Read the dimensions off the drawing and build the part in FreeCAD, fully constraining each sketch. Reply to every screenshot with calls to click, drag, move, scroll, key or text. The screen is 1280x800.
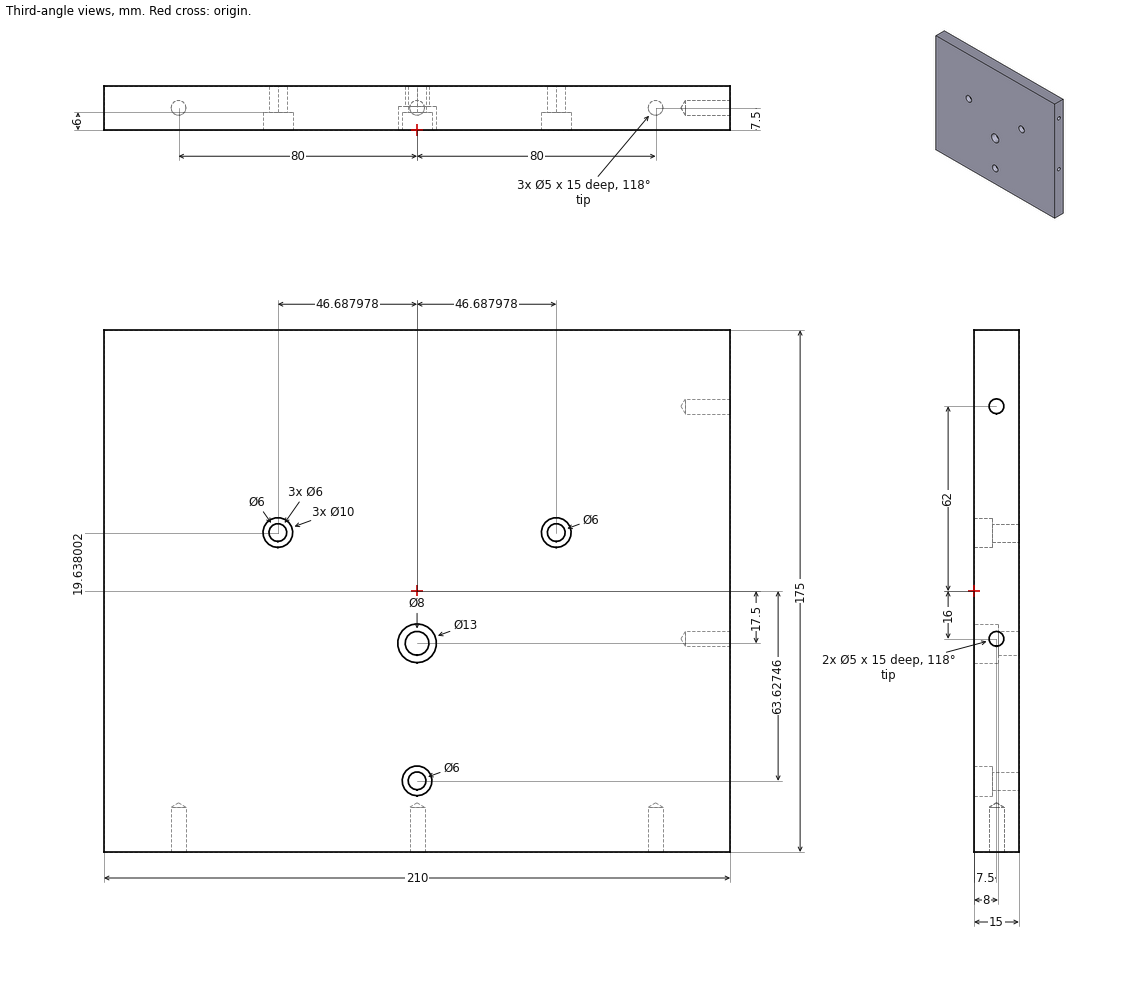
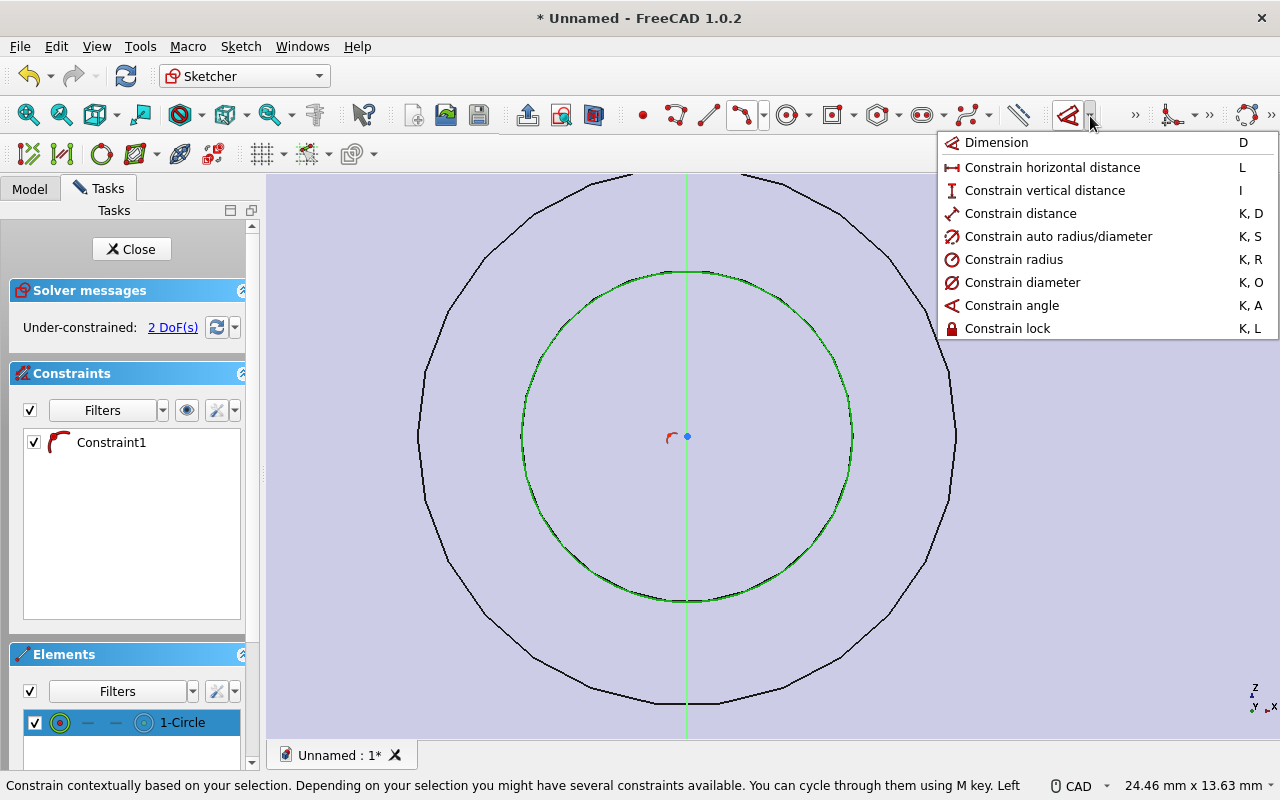
click(1108, 282)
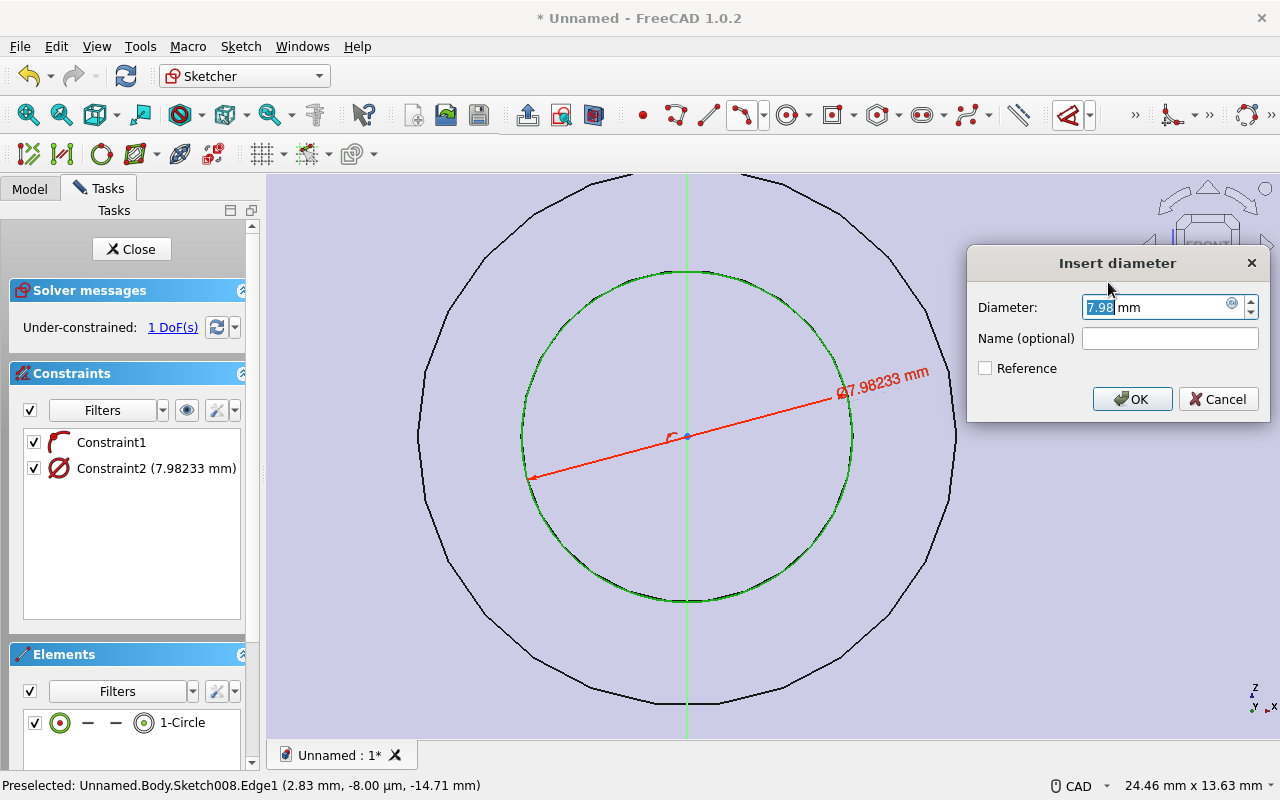
text(8)
key(Return)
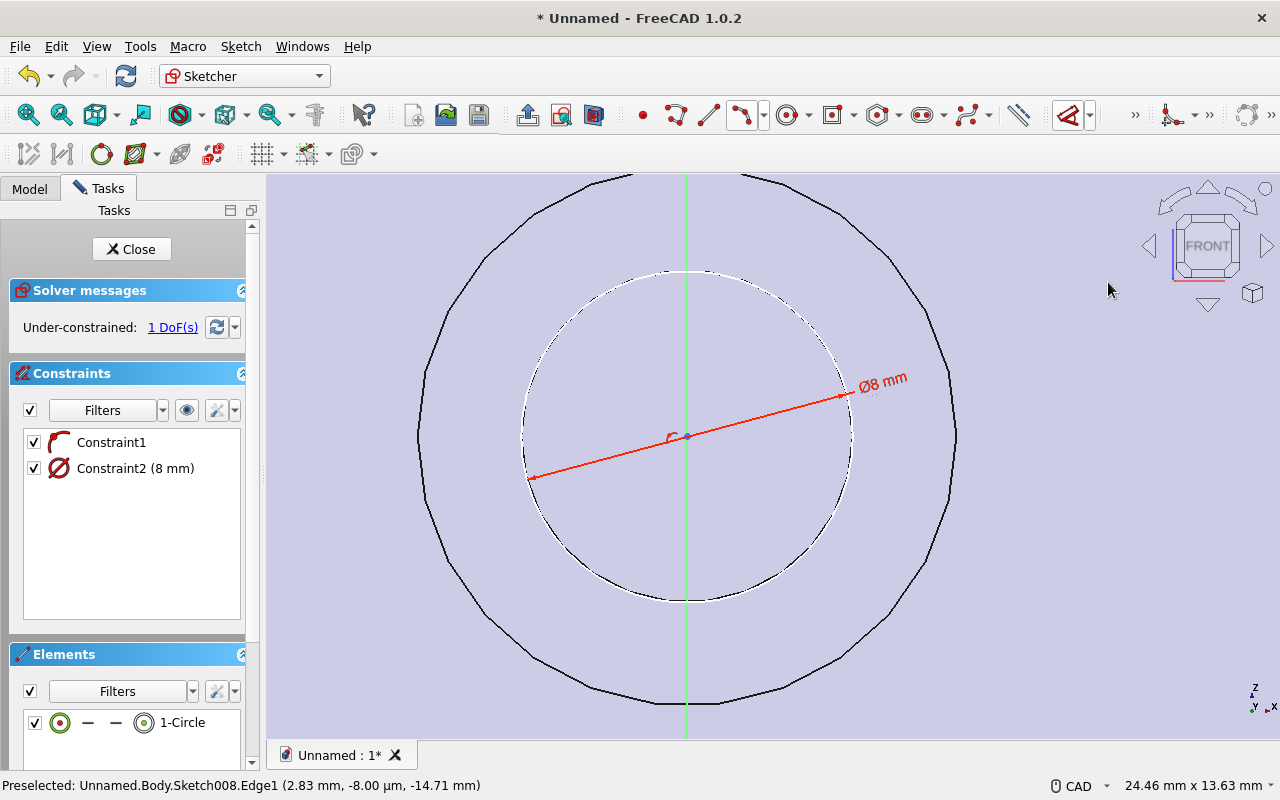
click(687, 437)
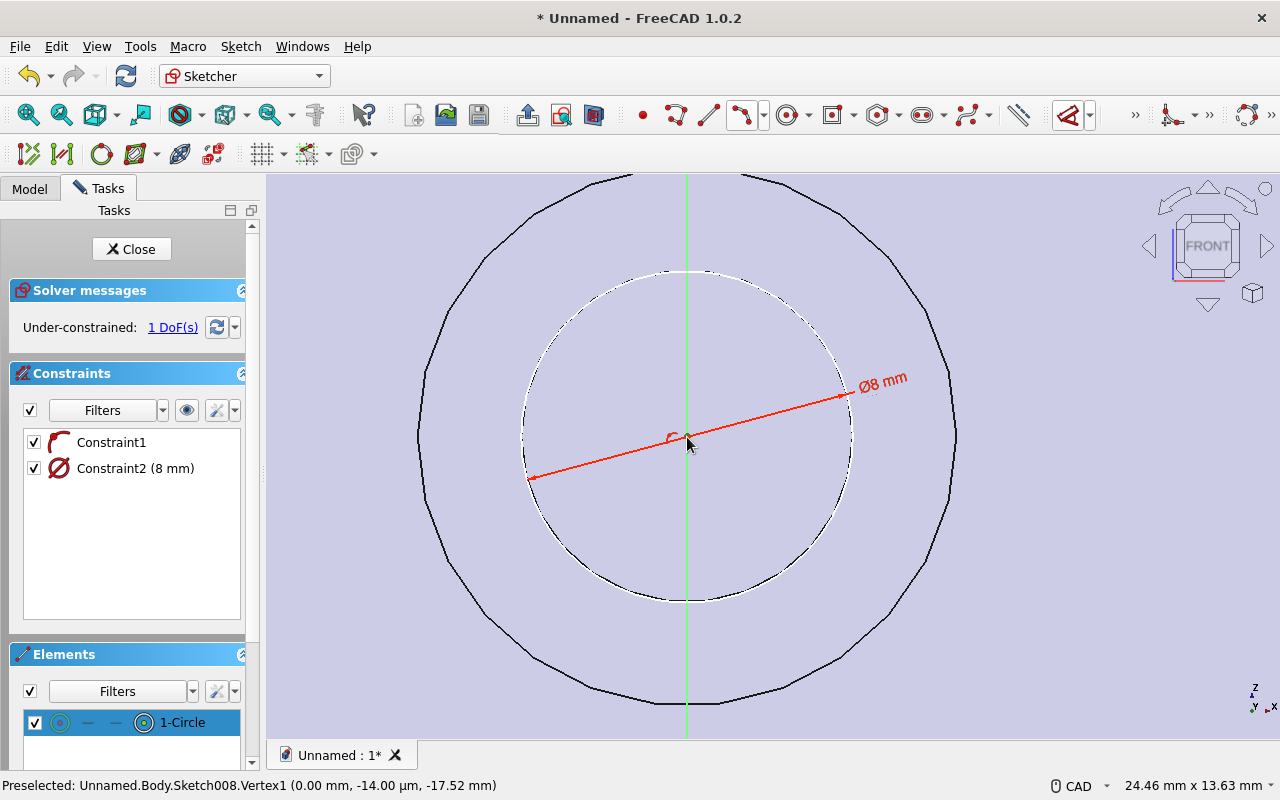
click(1090, 116)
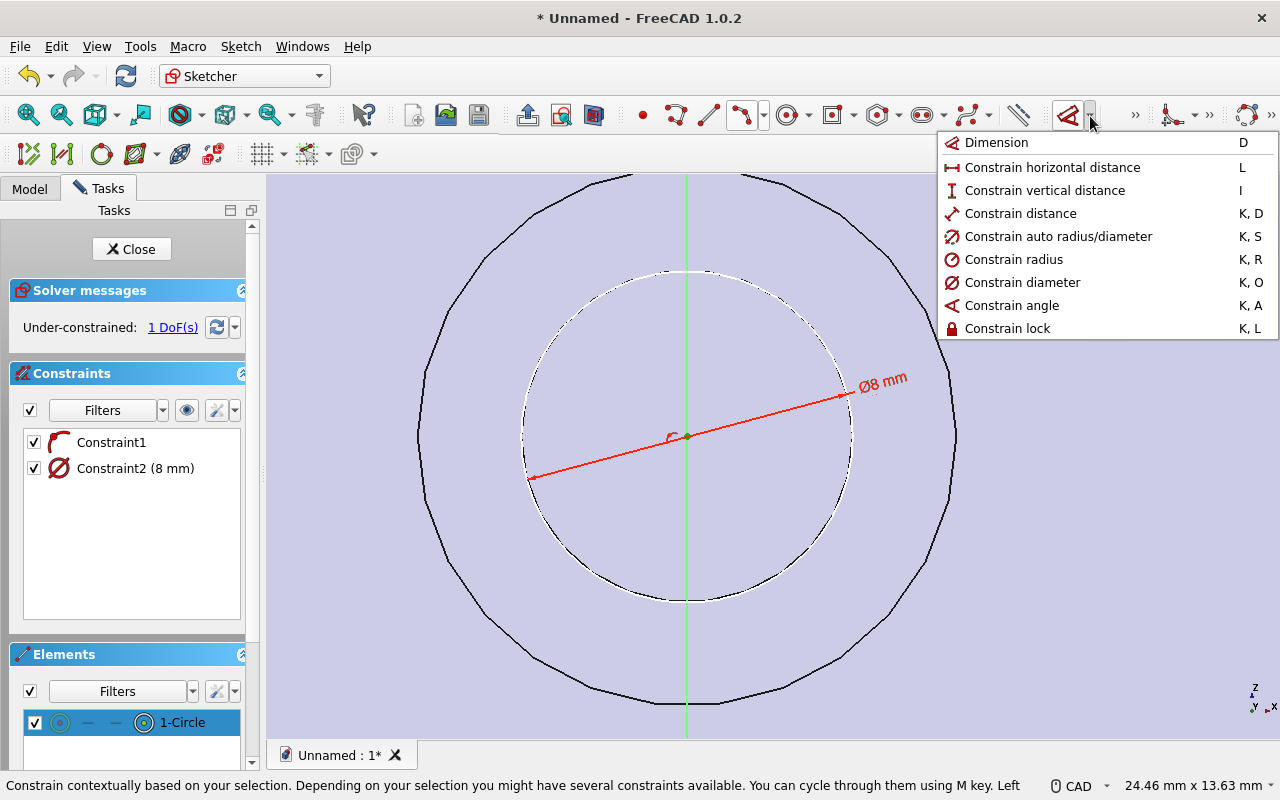
click(1108, 190)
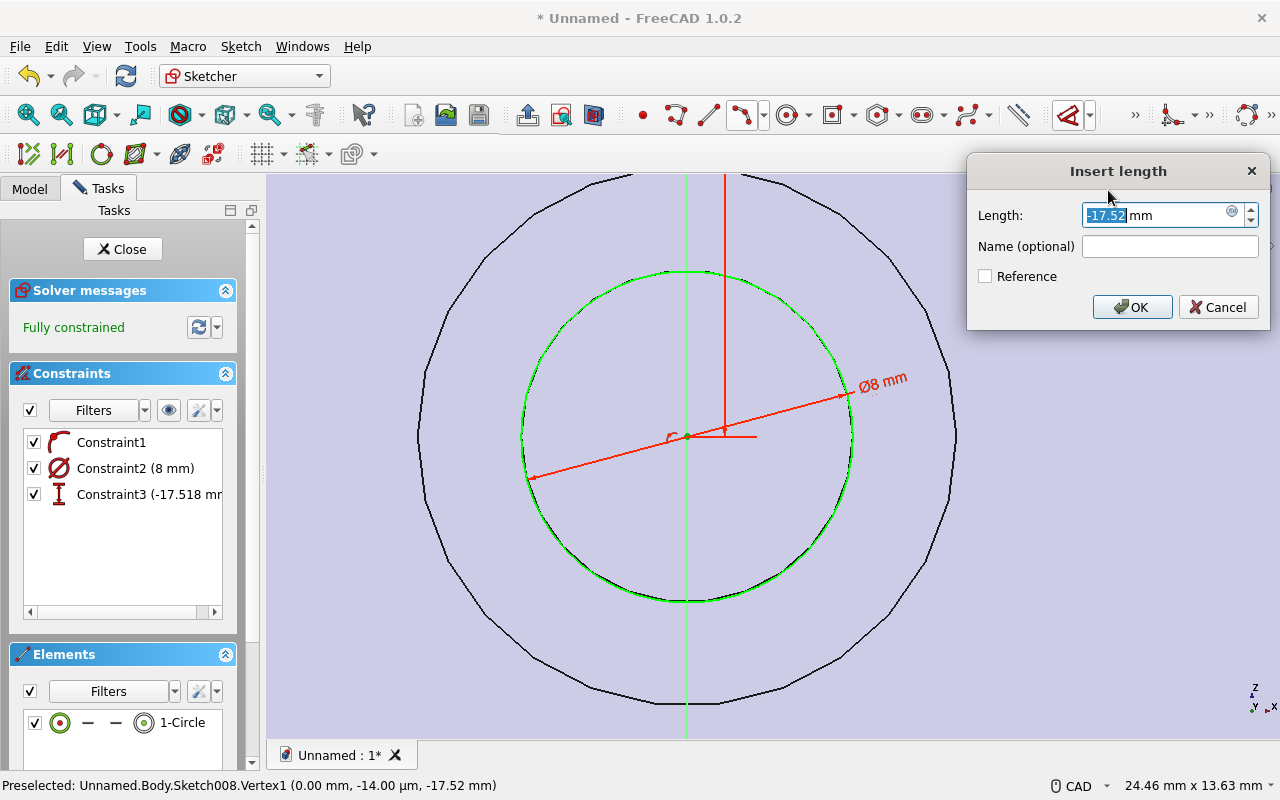
text(-17.5)
key(Return)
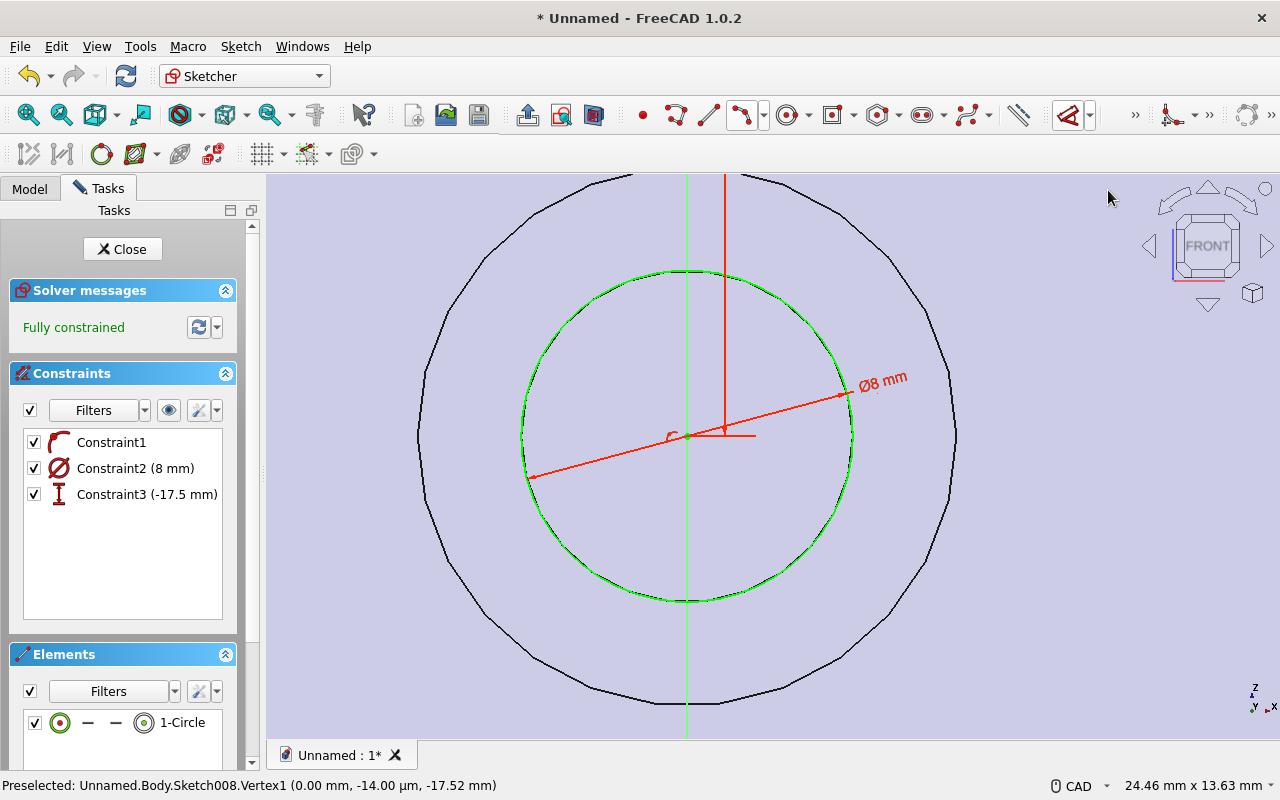
click(123, 249)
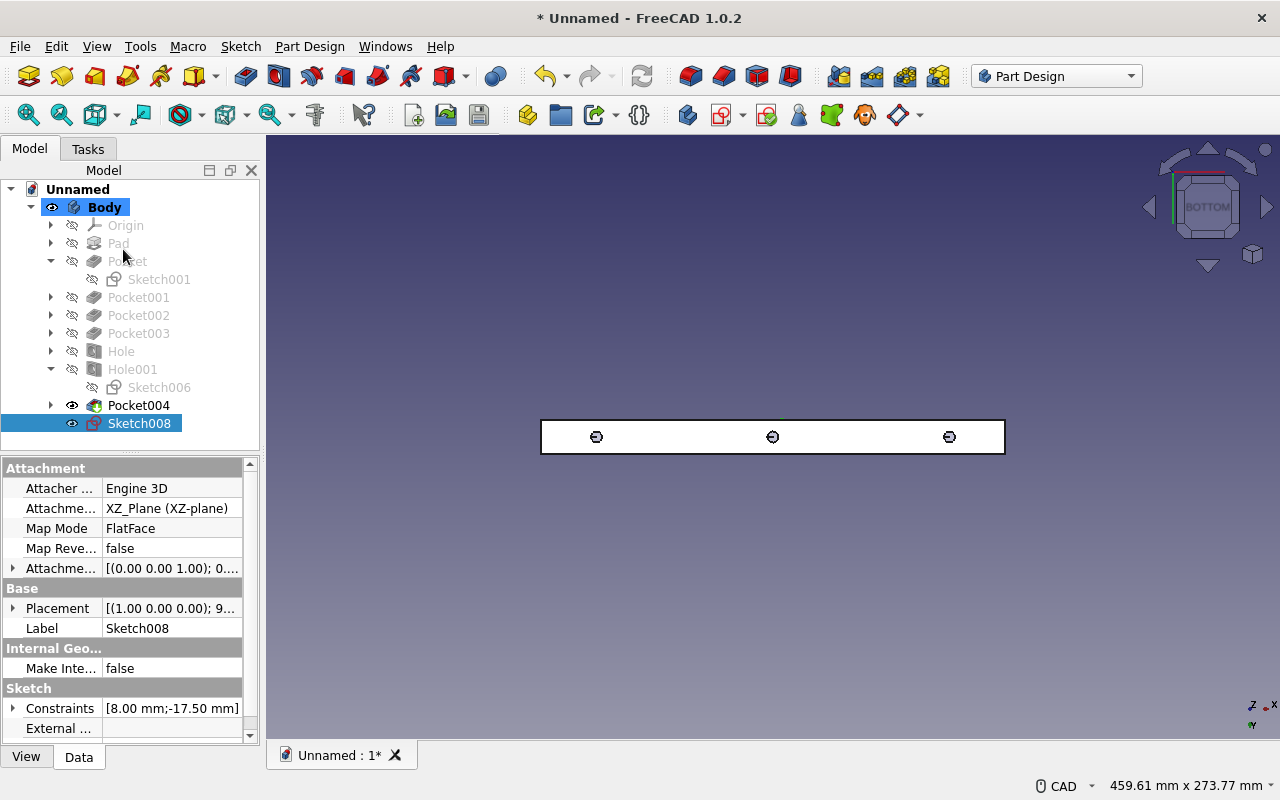
click(246, 76)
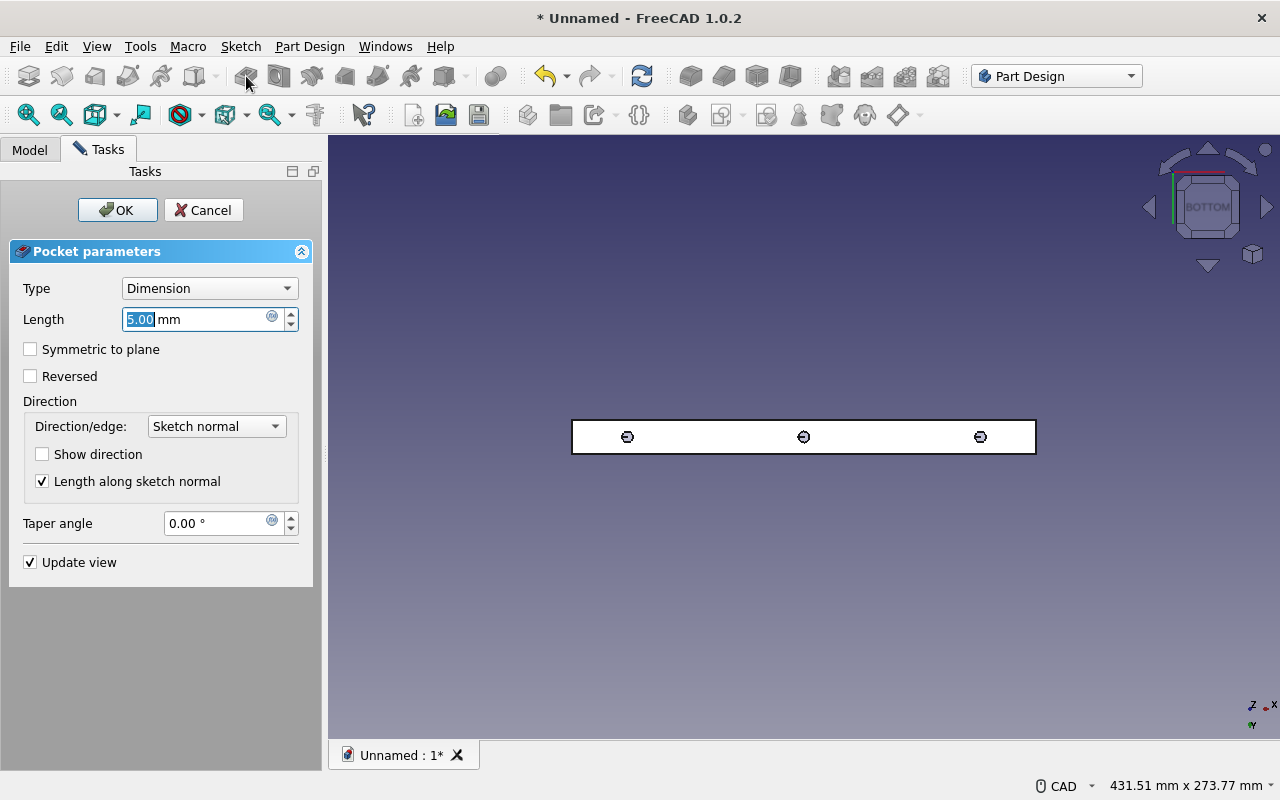
click(210, 288)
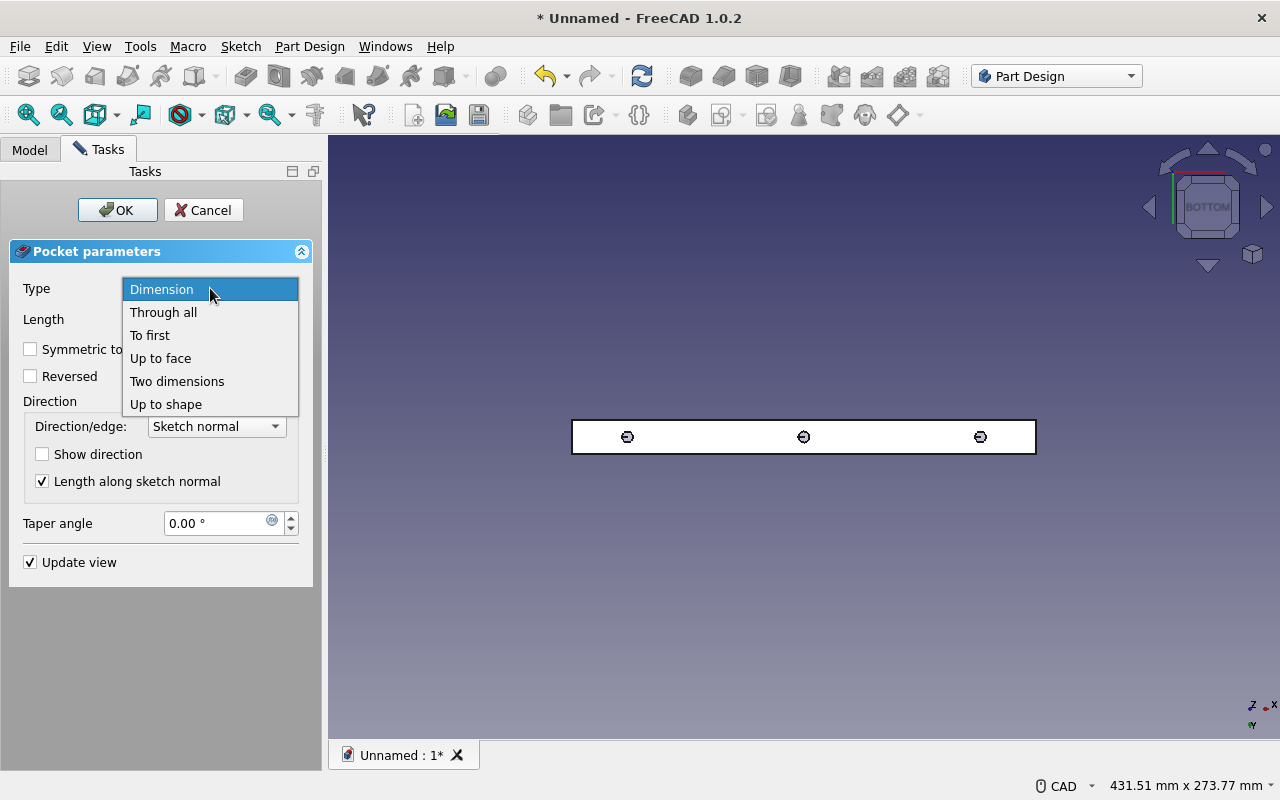
click(208, 336)